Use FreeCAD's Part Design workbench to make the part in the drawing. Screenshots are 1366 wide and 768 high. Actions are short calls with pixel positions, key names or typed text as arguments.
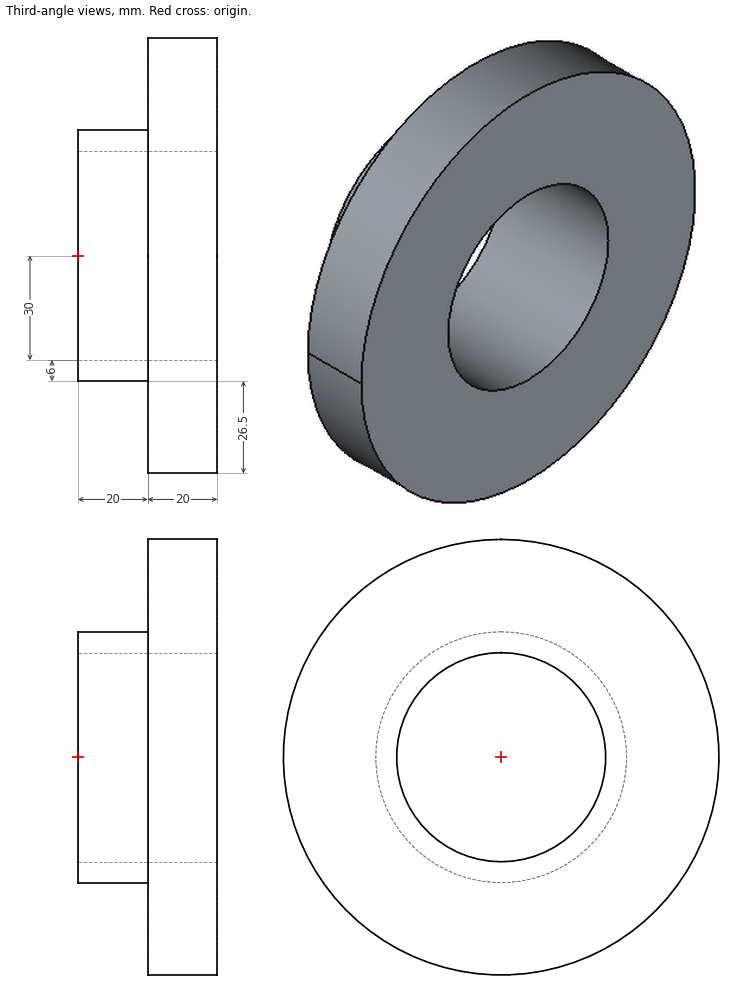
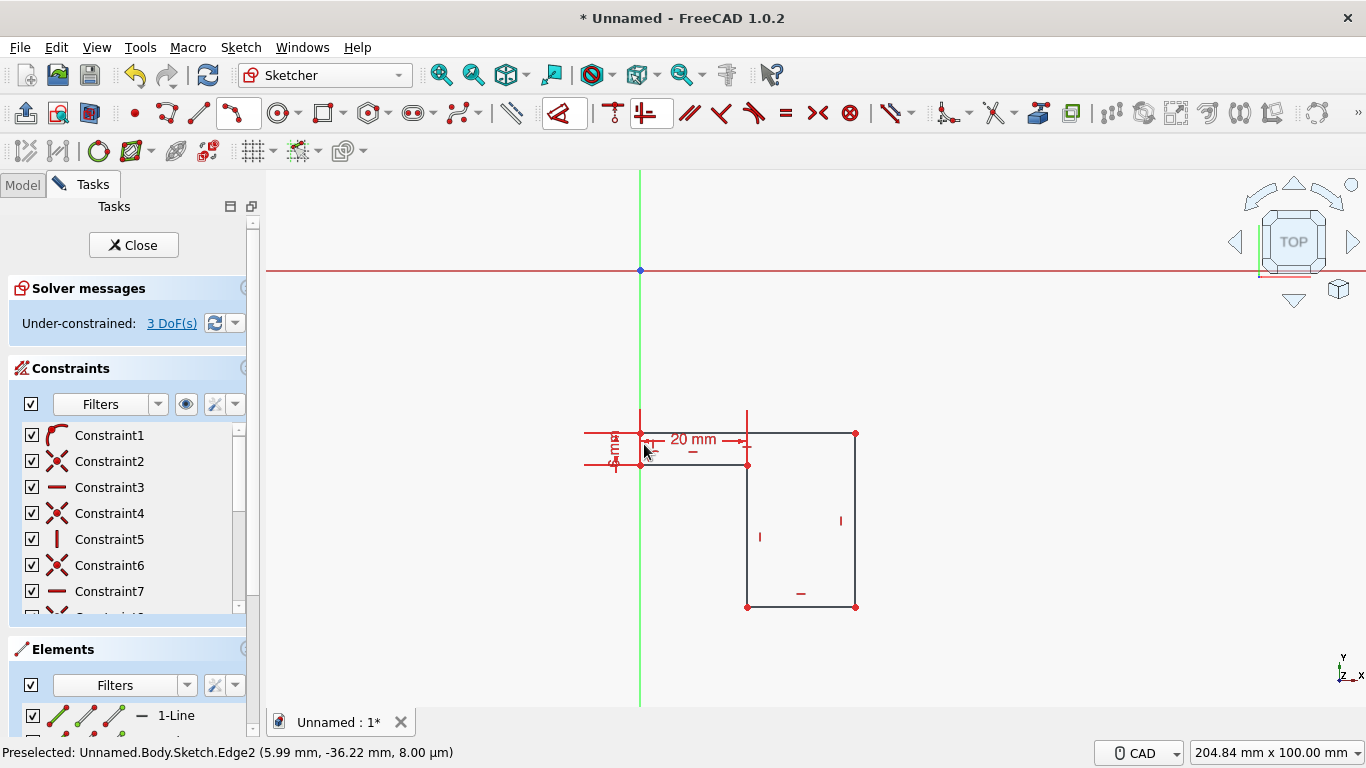
click(780, 607)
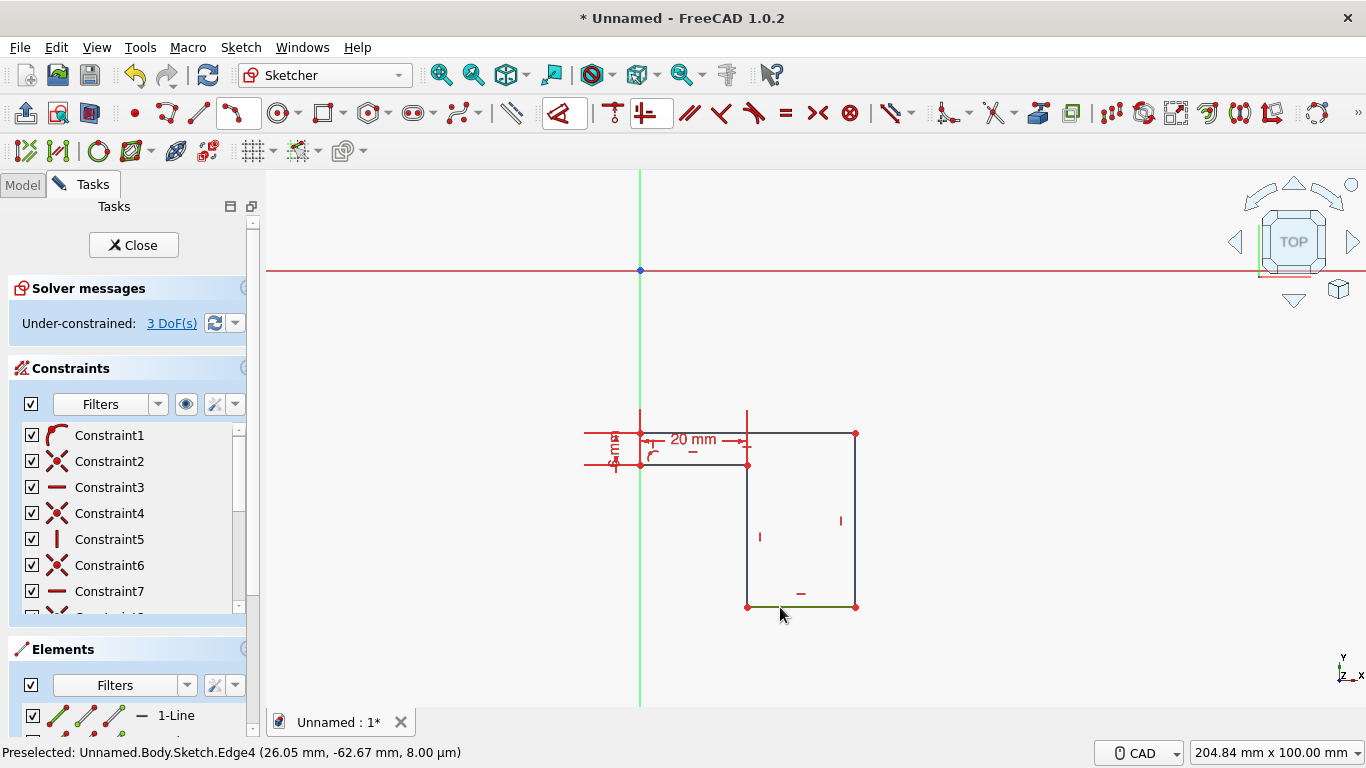
click(582, 114)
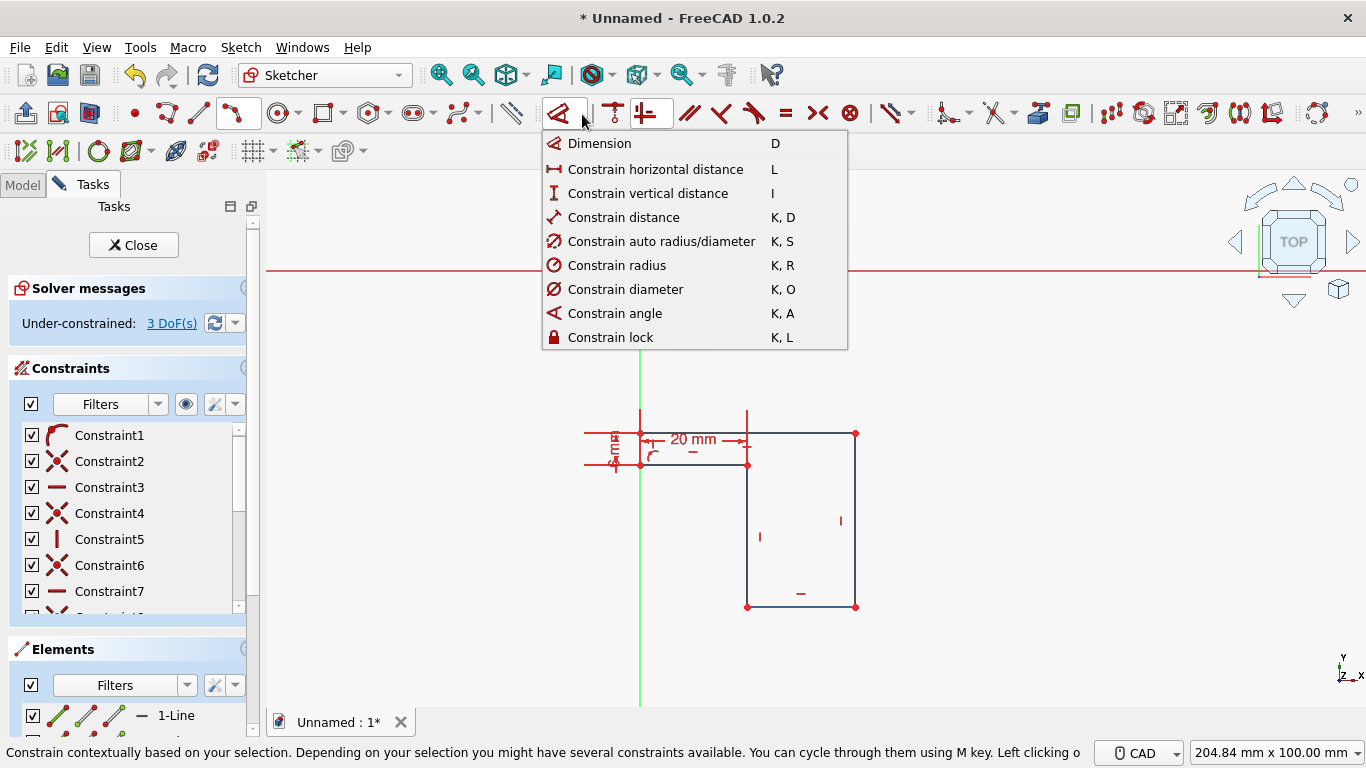
click(695, 169)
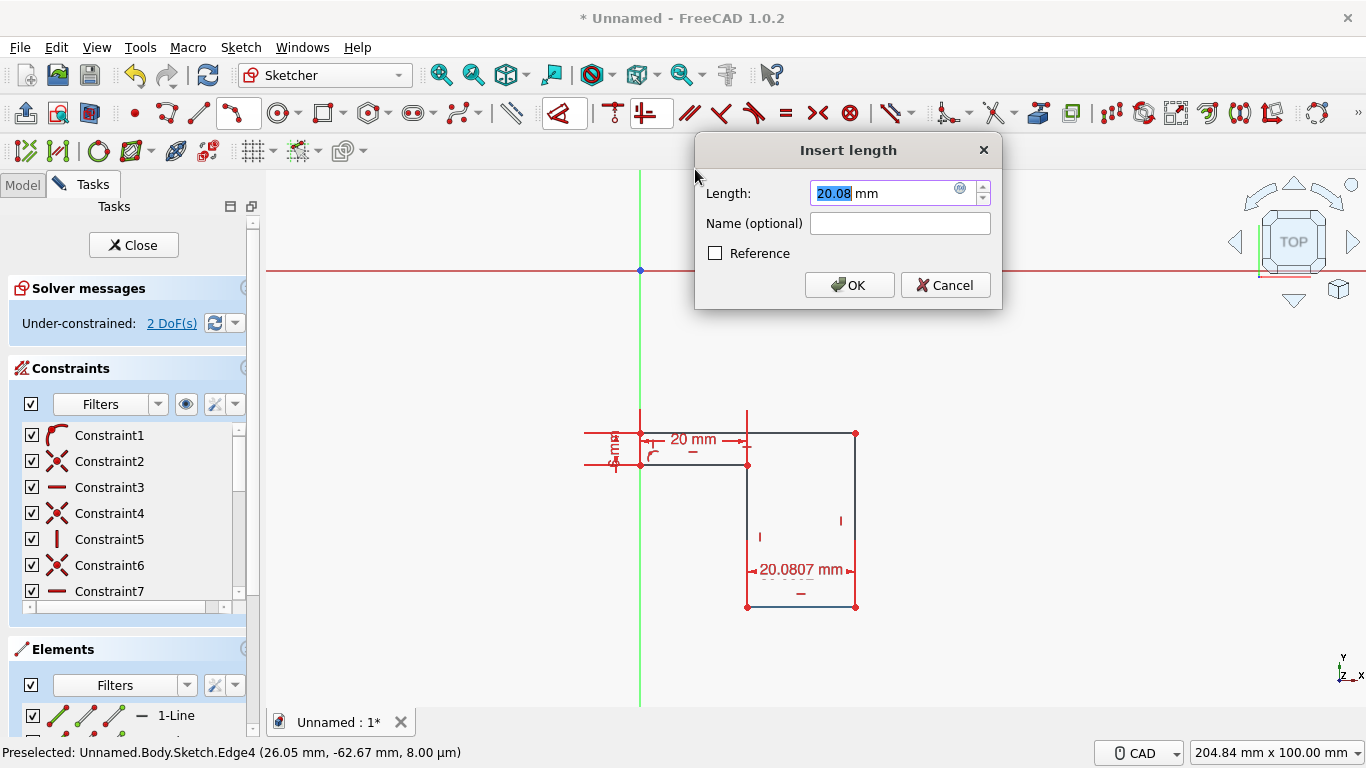
text(20)
key(Return)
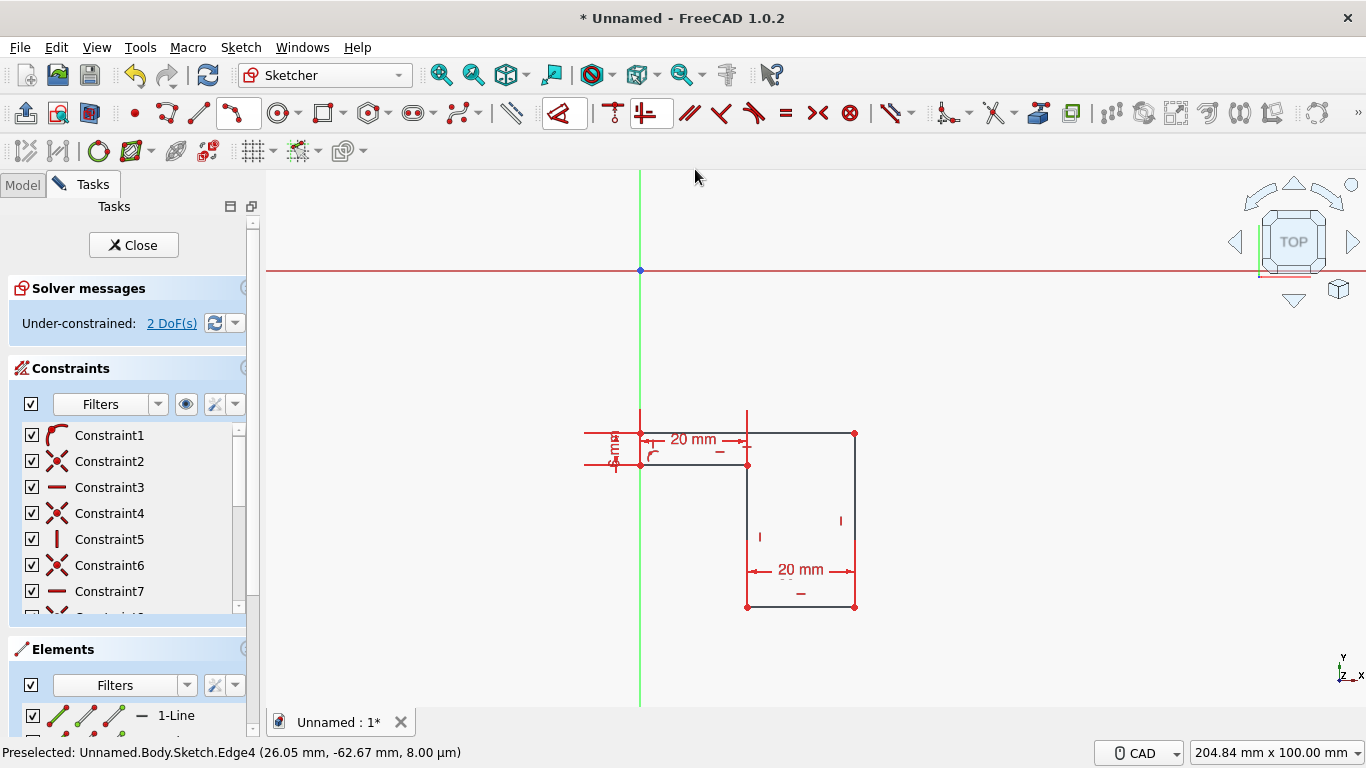
click(640, 433)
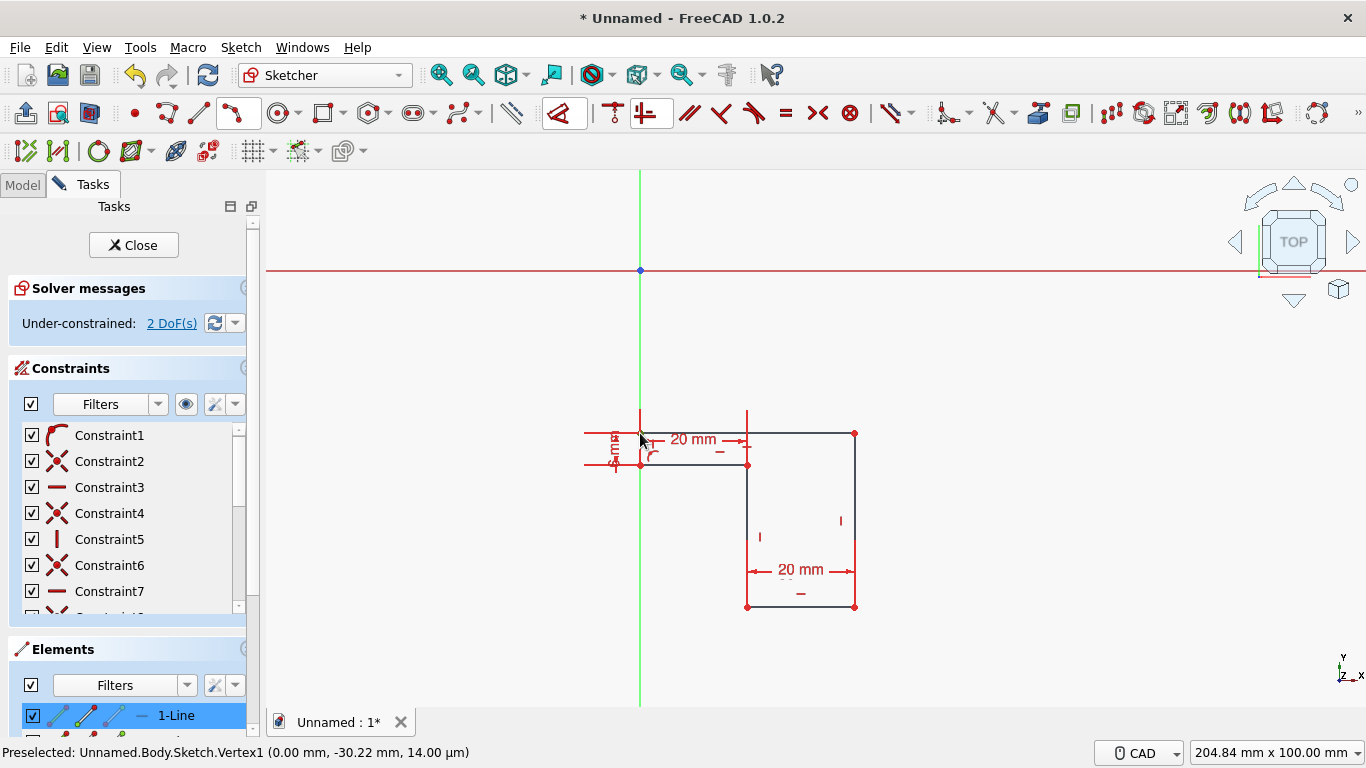
key(i)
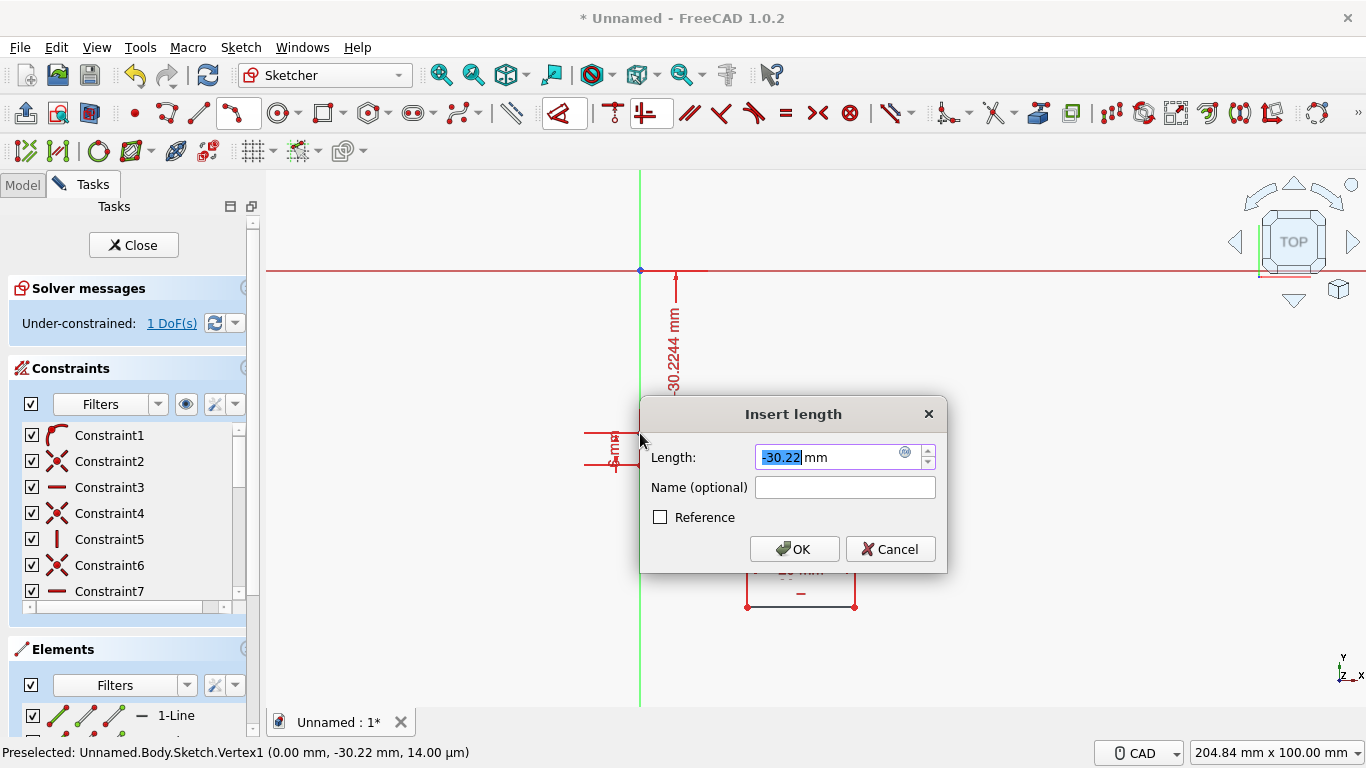
text(-30)
key(Return)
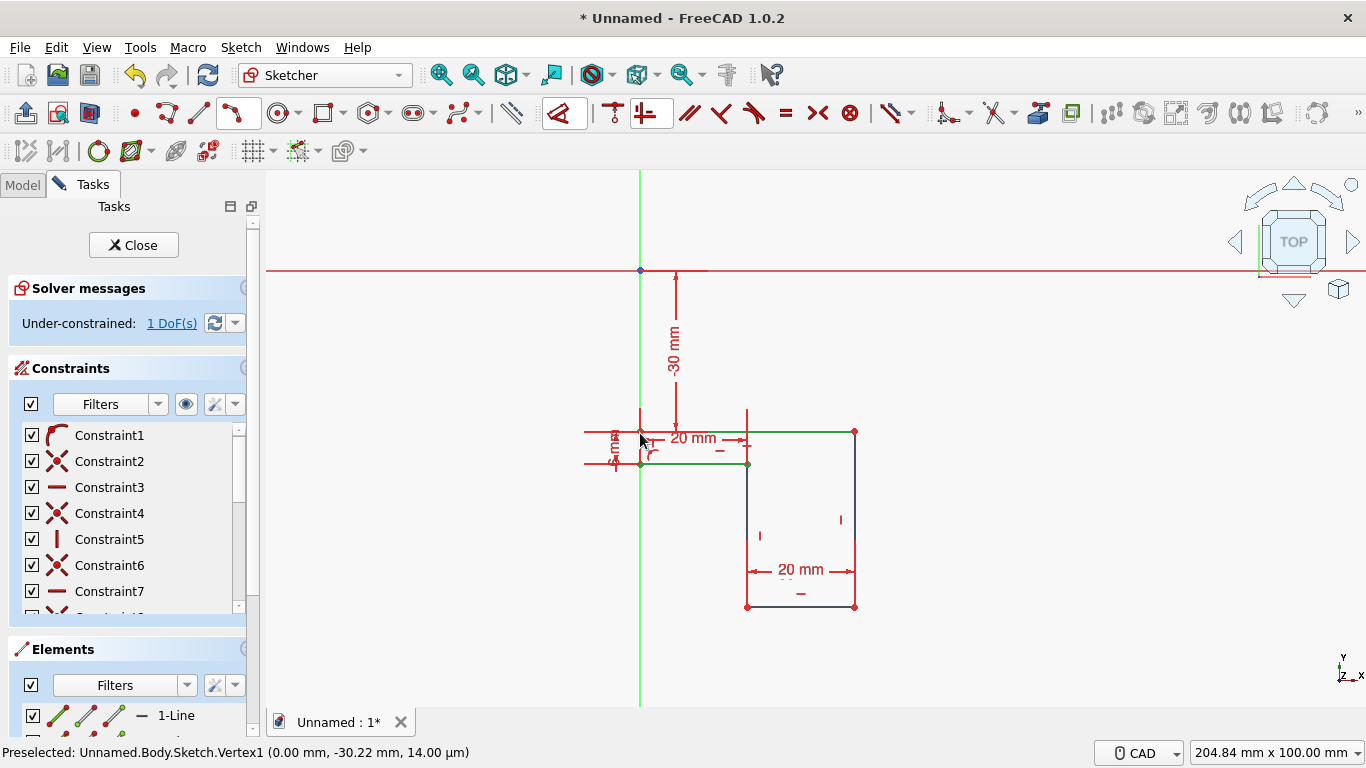
click(747, 507)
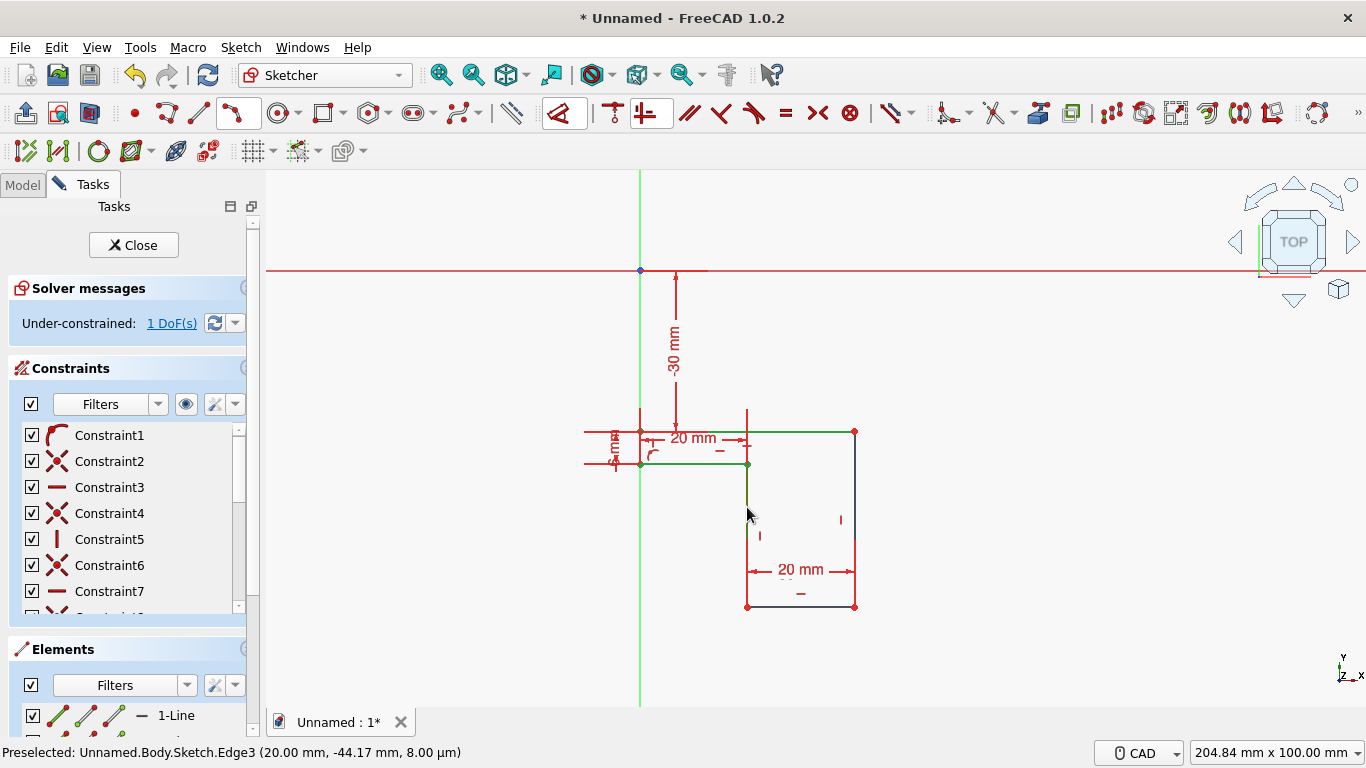
click(582, 114)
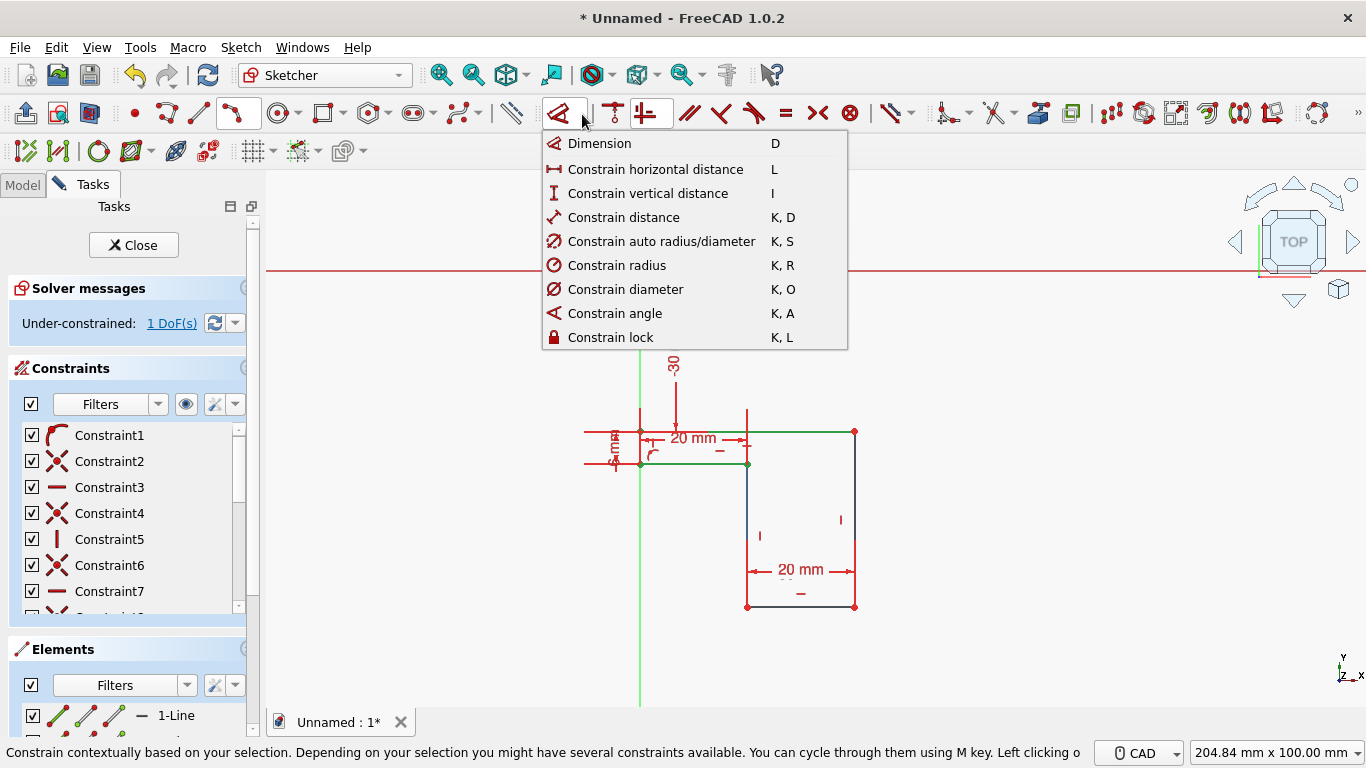
click(695, 193)